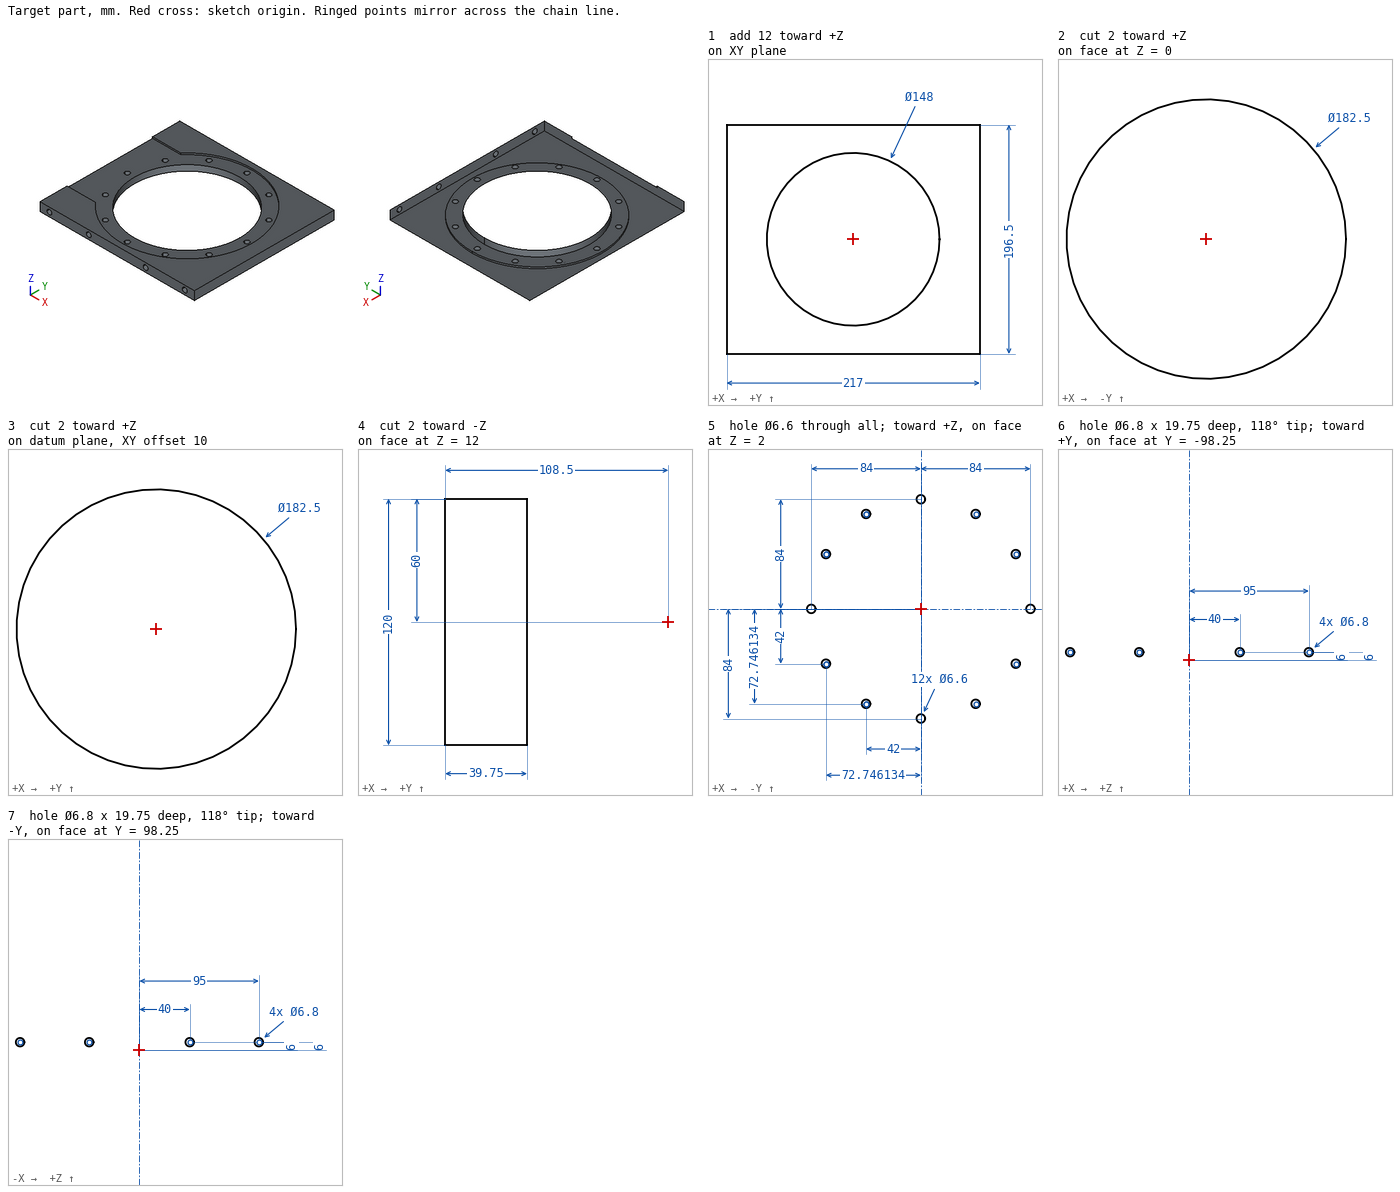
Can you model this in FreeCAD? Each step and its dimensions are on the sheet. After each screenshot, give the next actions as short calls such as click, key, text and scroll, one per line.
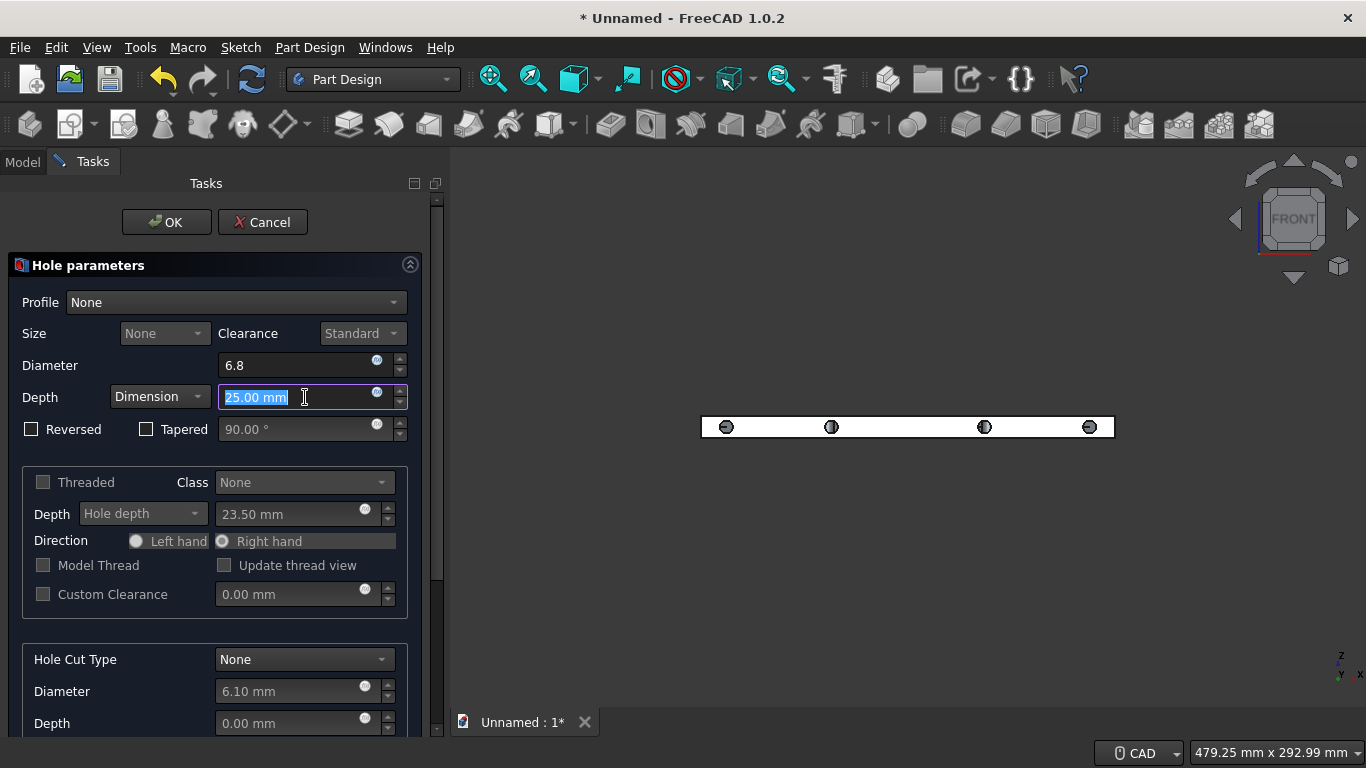
text(19.75)
key(Tab)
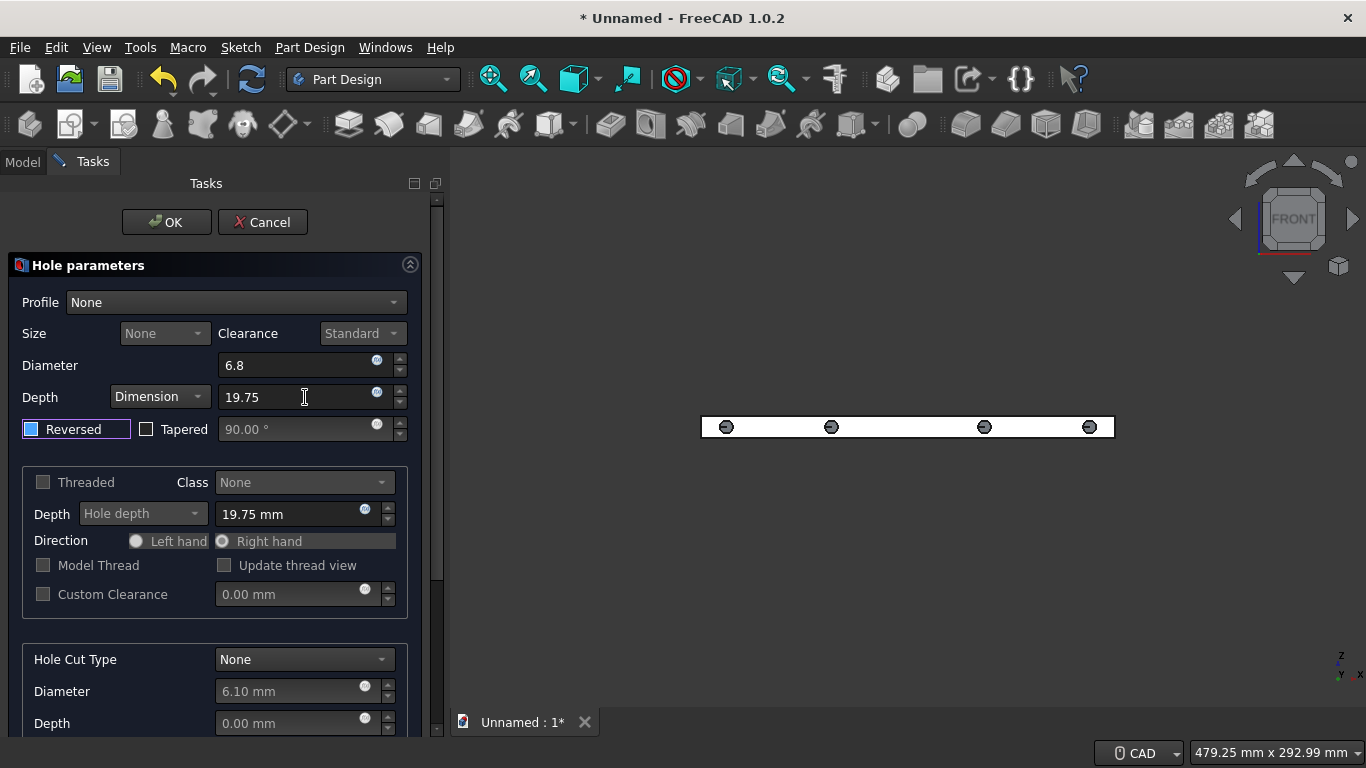
click(167, 222)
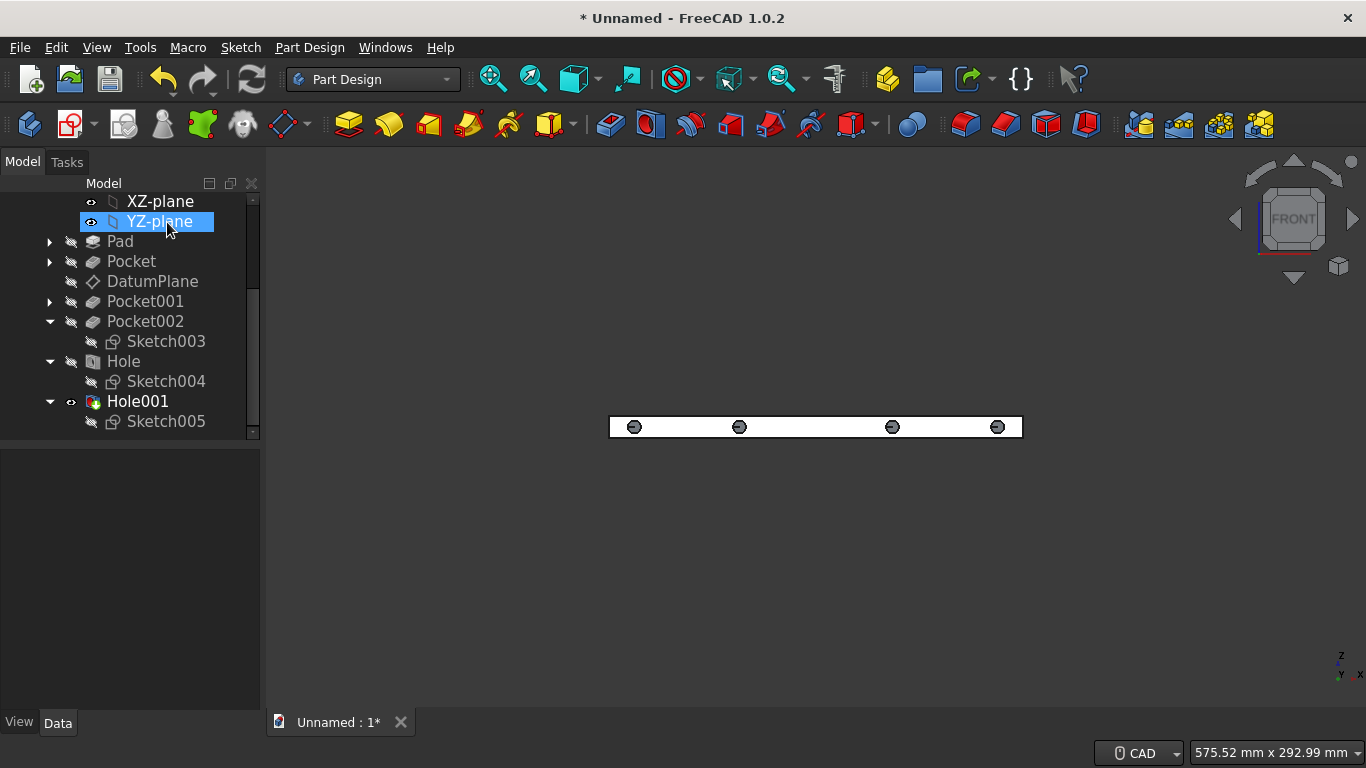
click(494, 80)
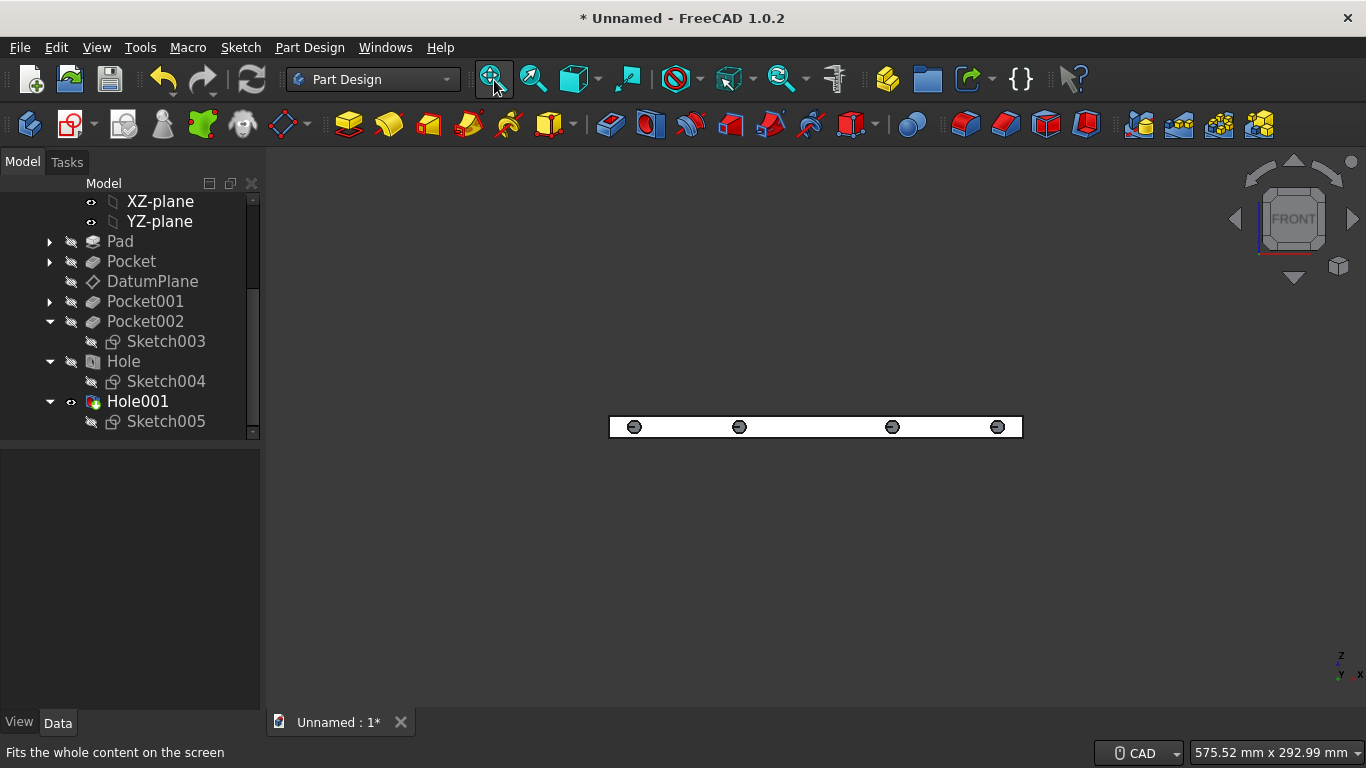
key(4)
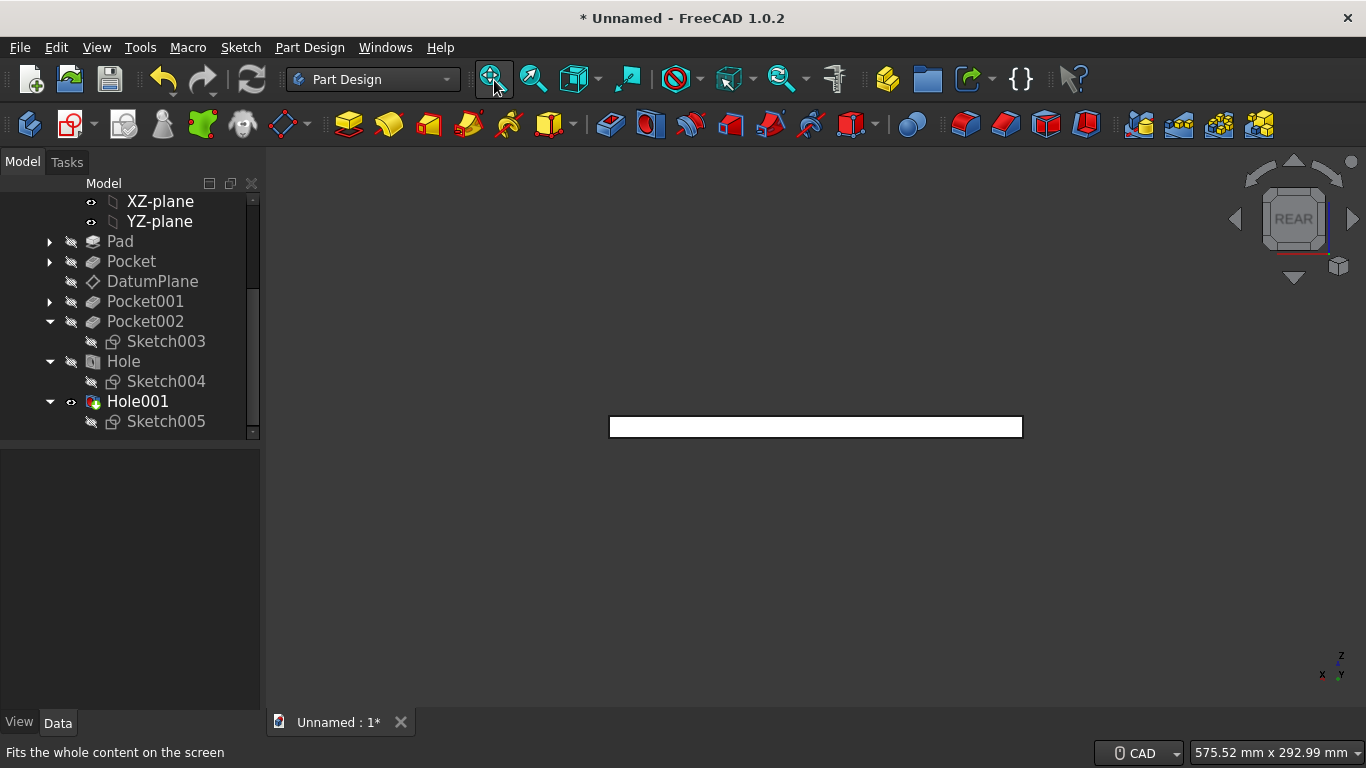
click(494, 80)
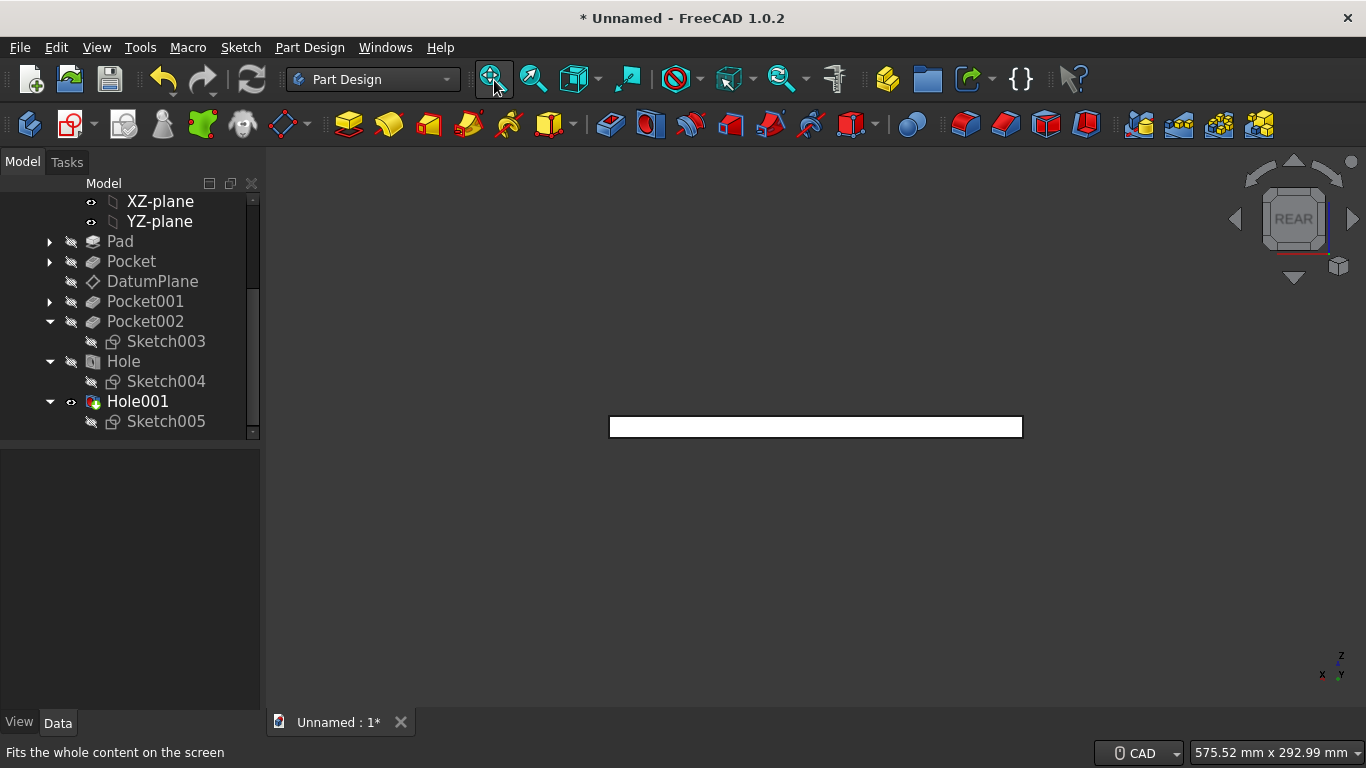
click(638, 426)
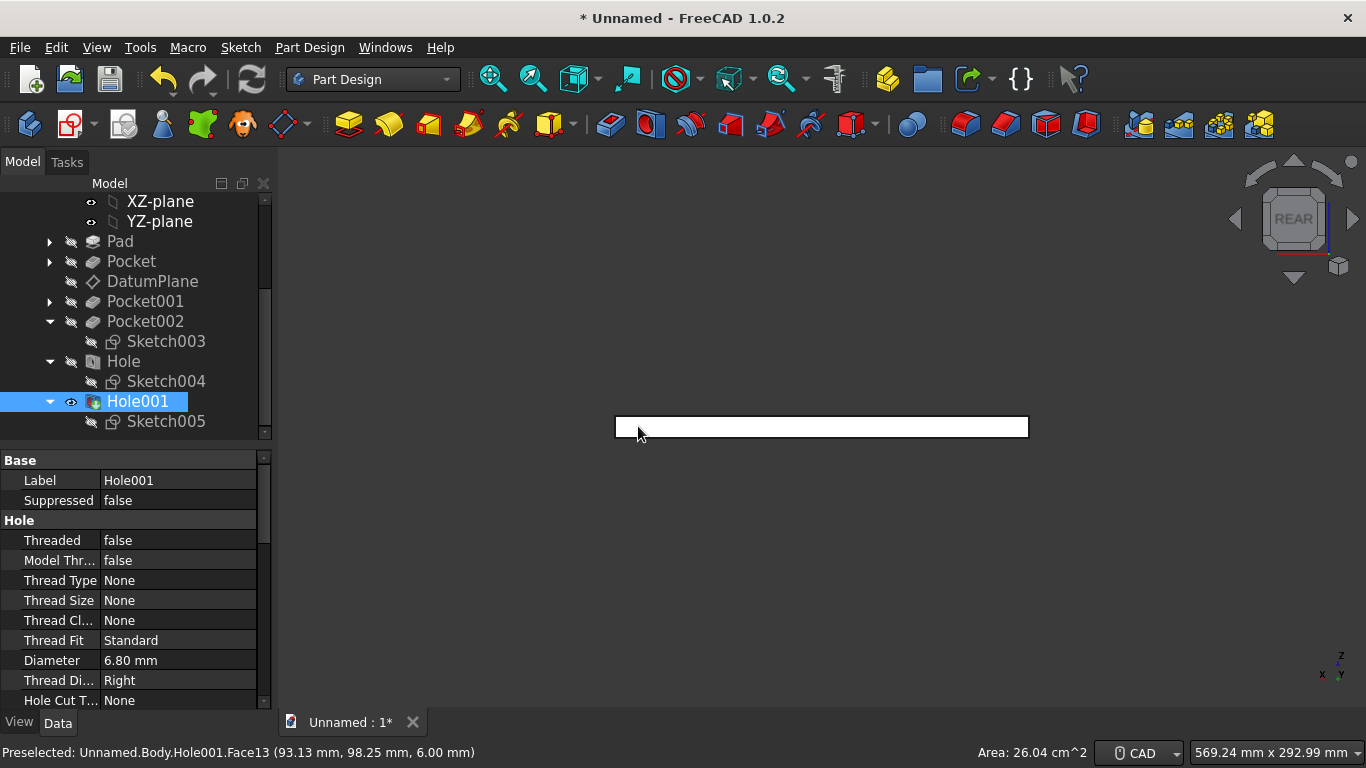
click(70, 124)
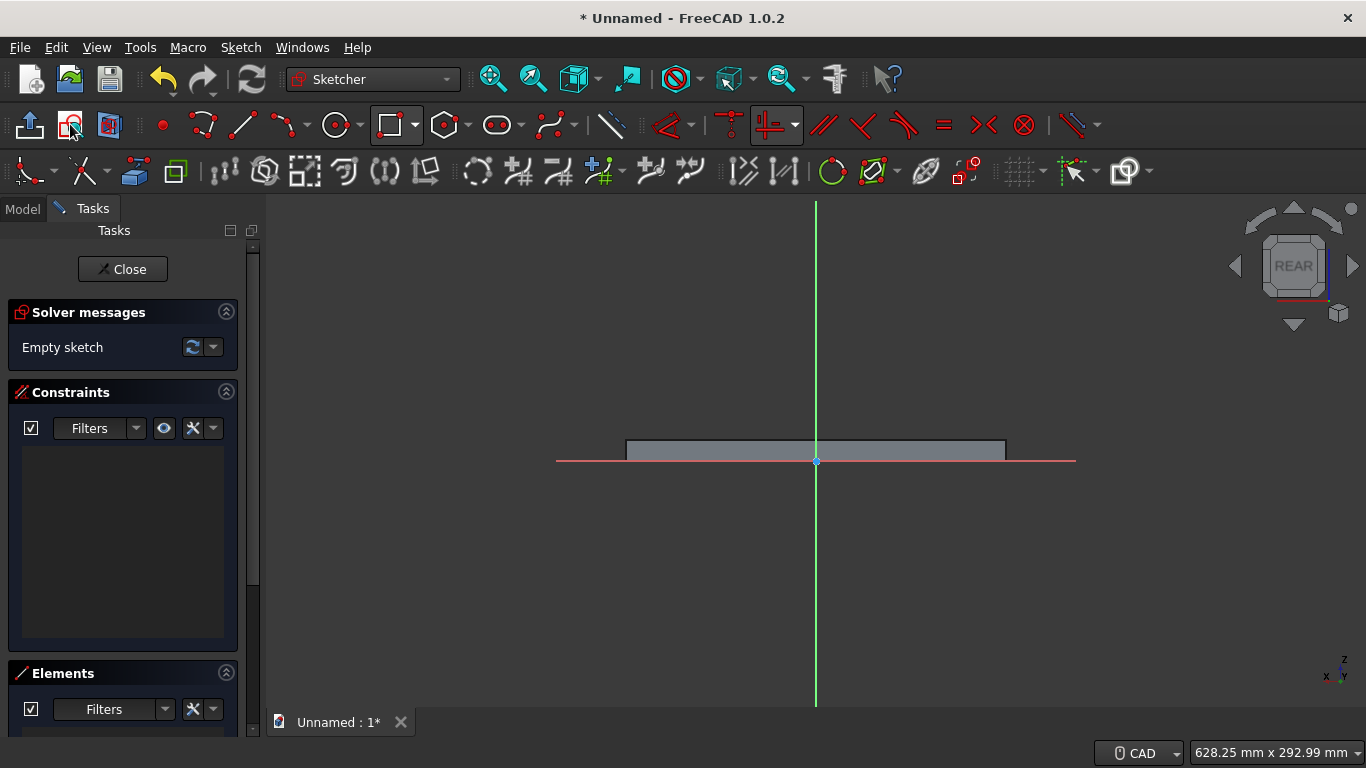
scroll(899, 456, up, 3)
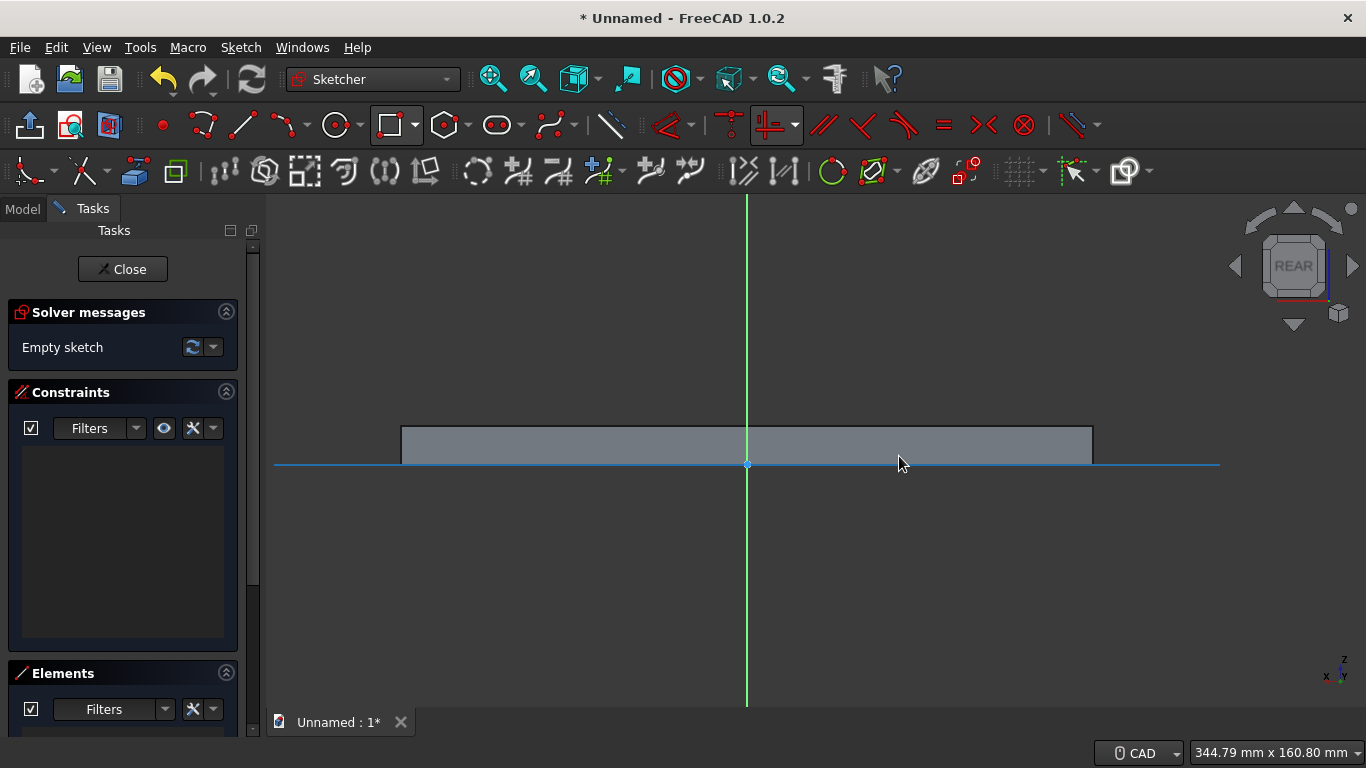
click(336, 126)